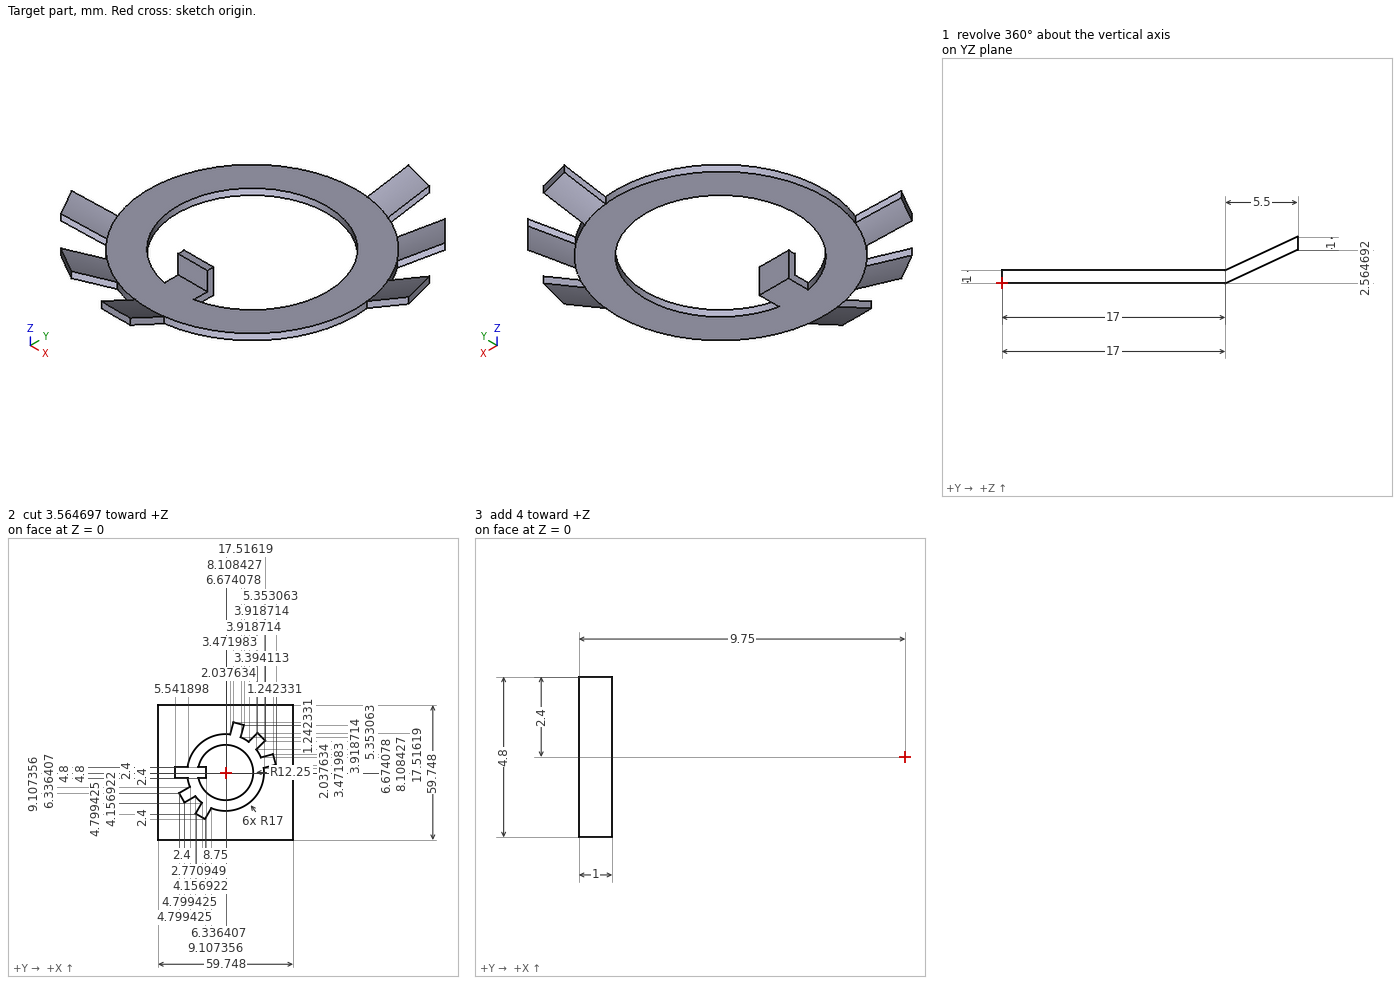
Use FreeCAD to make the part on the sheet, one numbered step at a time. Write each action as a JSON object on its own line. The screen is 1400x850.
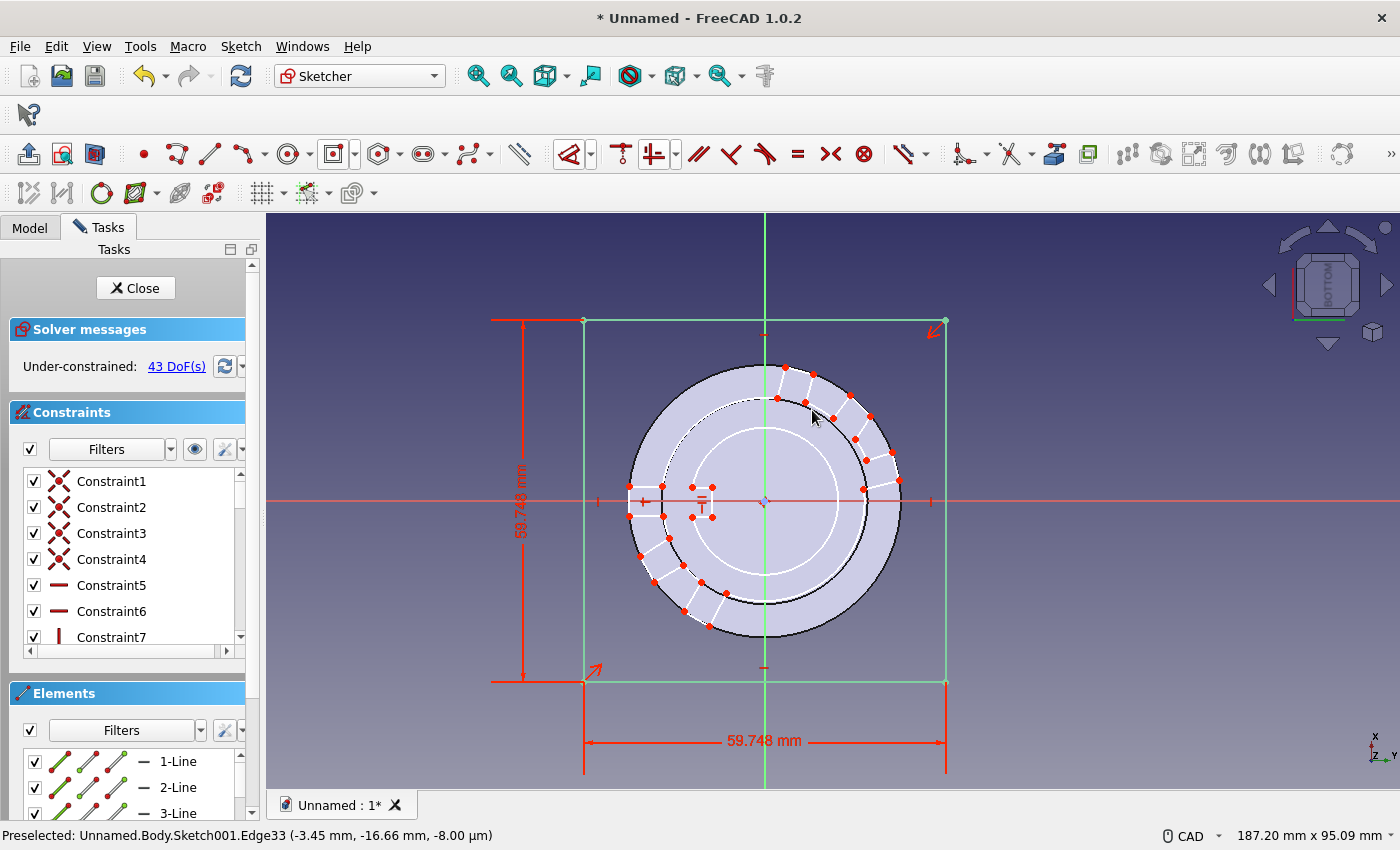
{"action": "scroll", "coordinate": [689, 571], "scroll_direction": "up", "scroll_amount": 4}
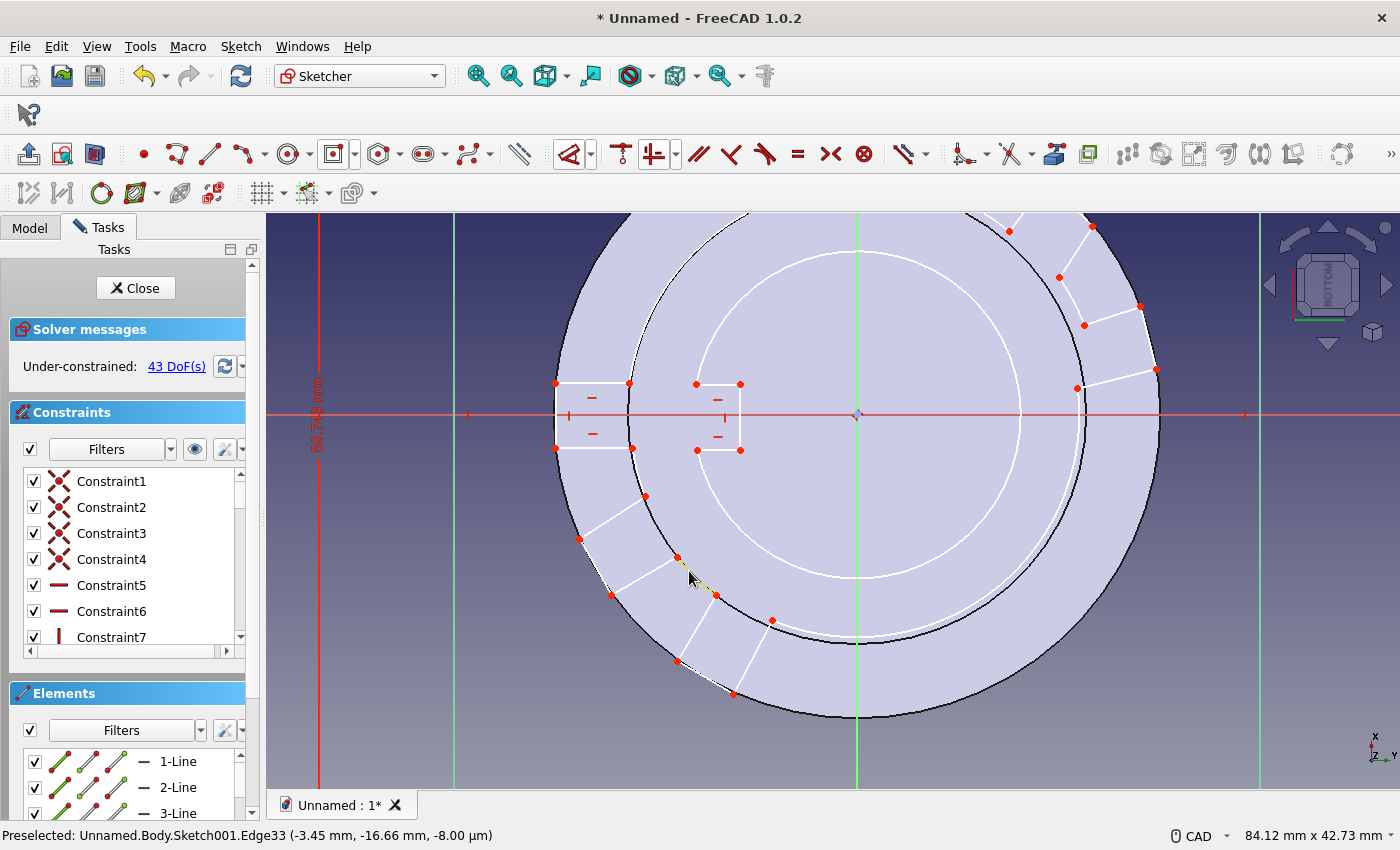
{"action": "left_click", "coordinate": [688, 570]}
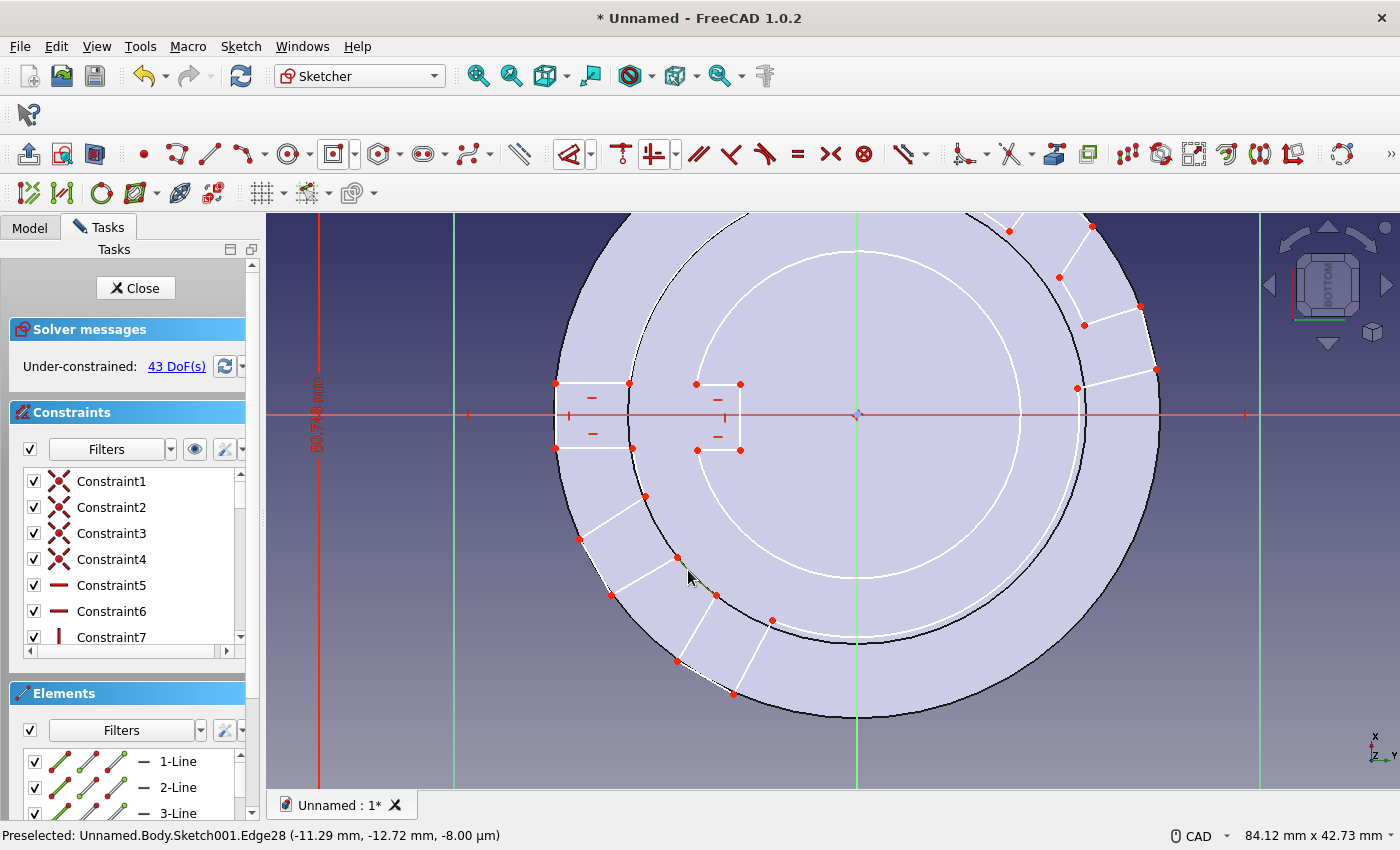
{"action": "left_click", "coordinate": [908, 631]}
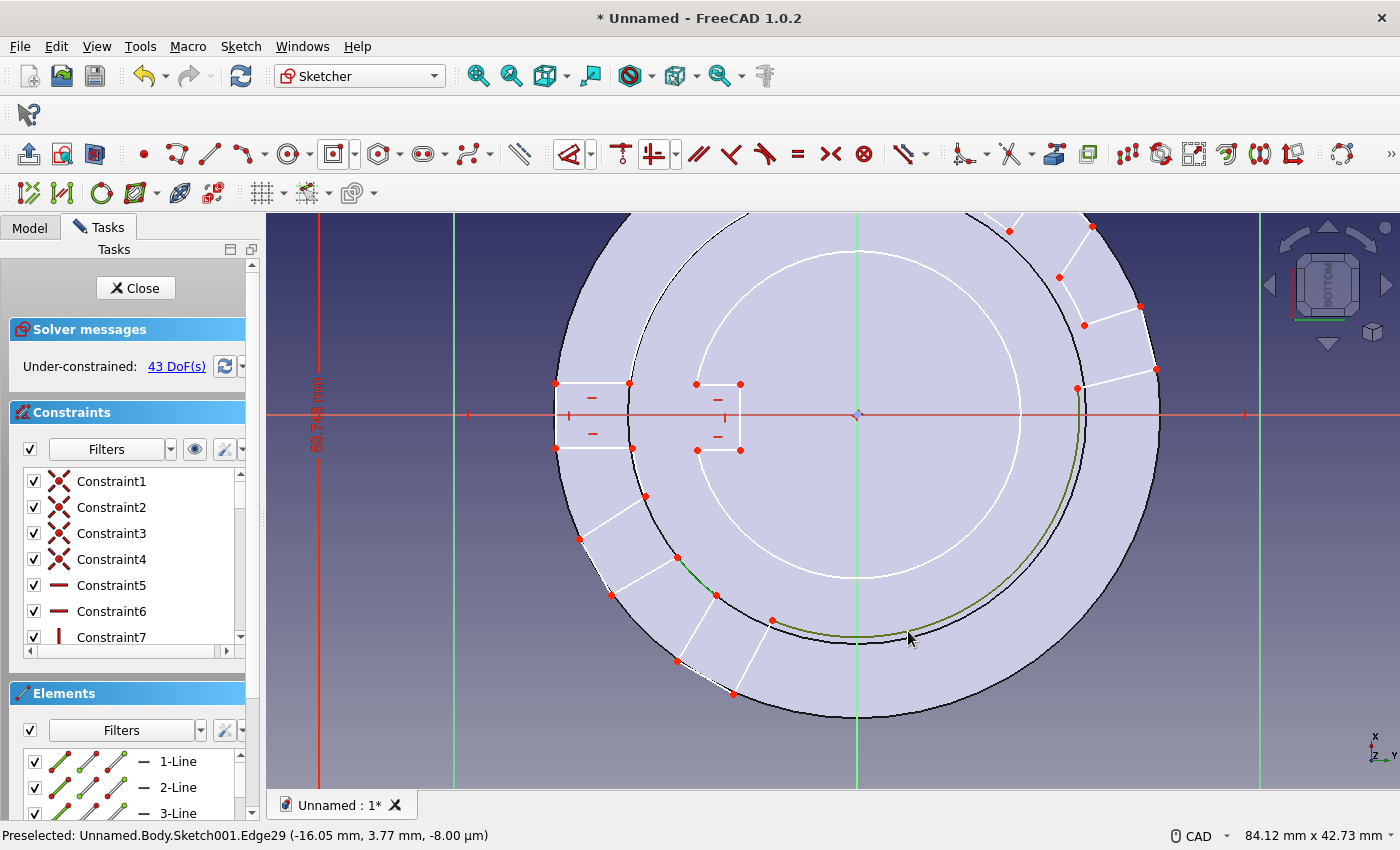
{"action": "left_click", "coordinate": [1078, 310]}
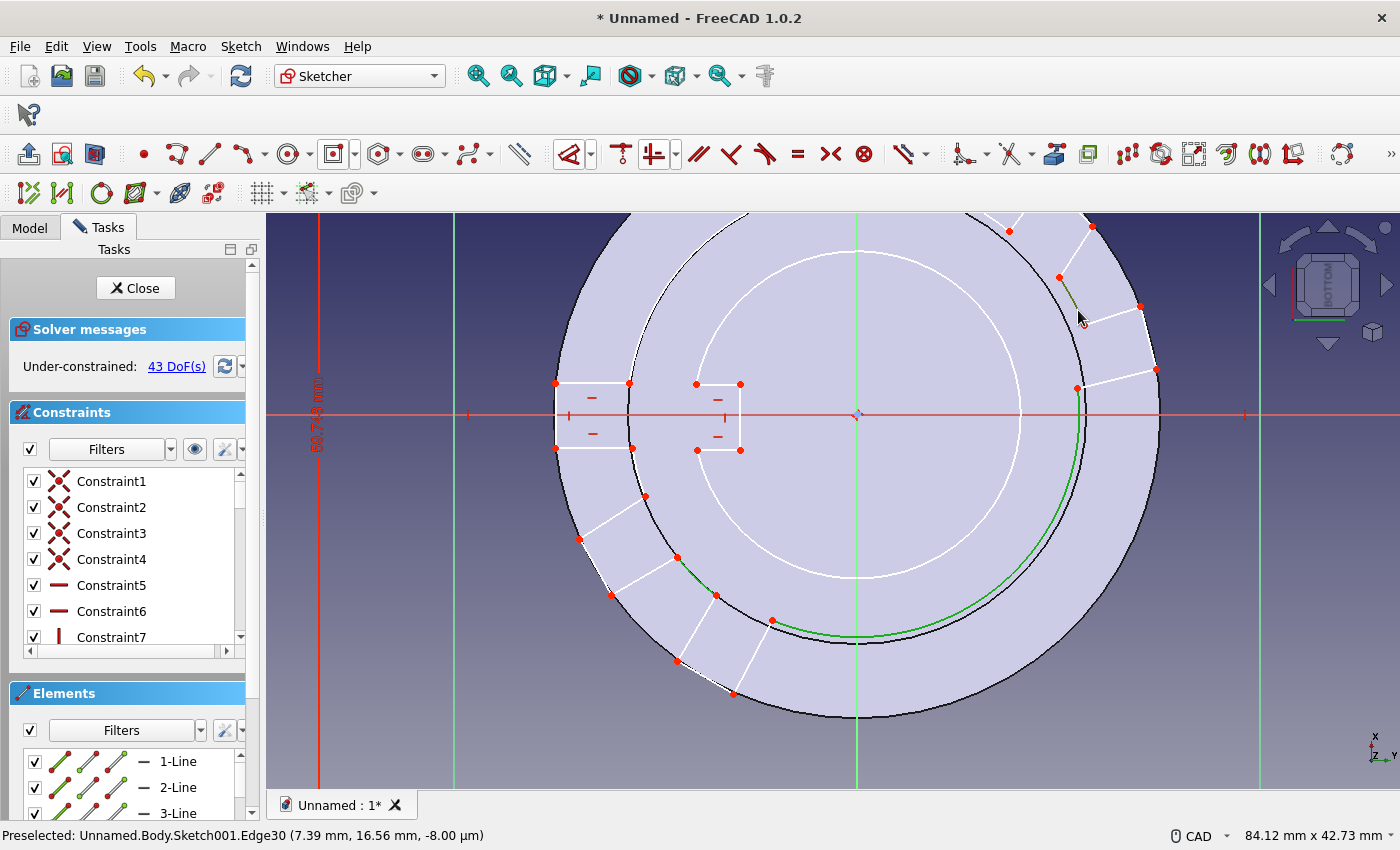
{"action": "scroll", "coordinate": [689, 571], "scroll_direction": "down", "scroll_amount": 4}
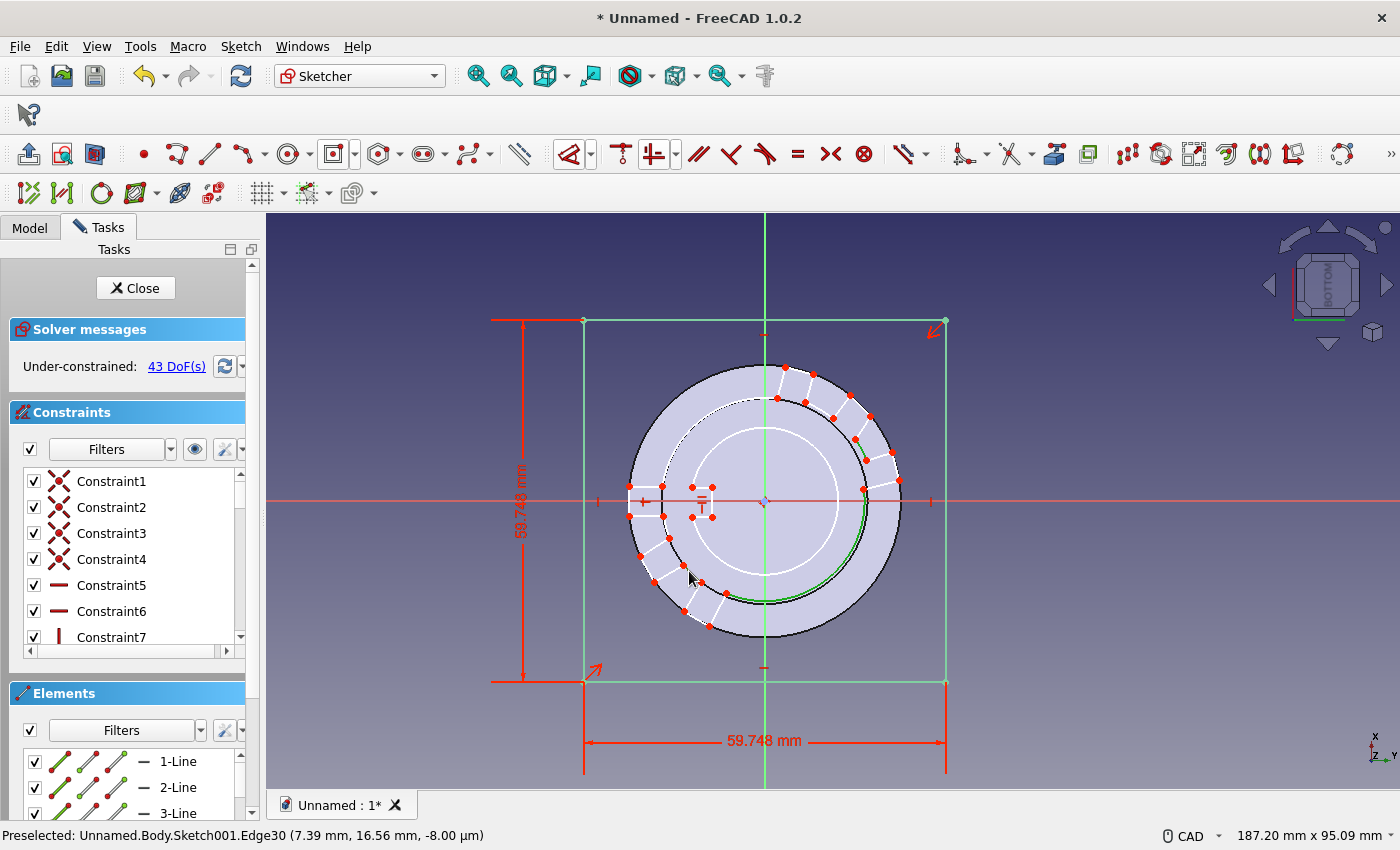
{"action": "scroll", "coordinate": [826, 413], "scroll_direction": "up", "scroll_amount": 2}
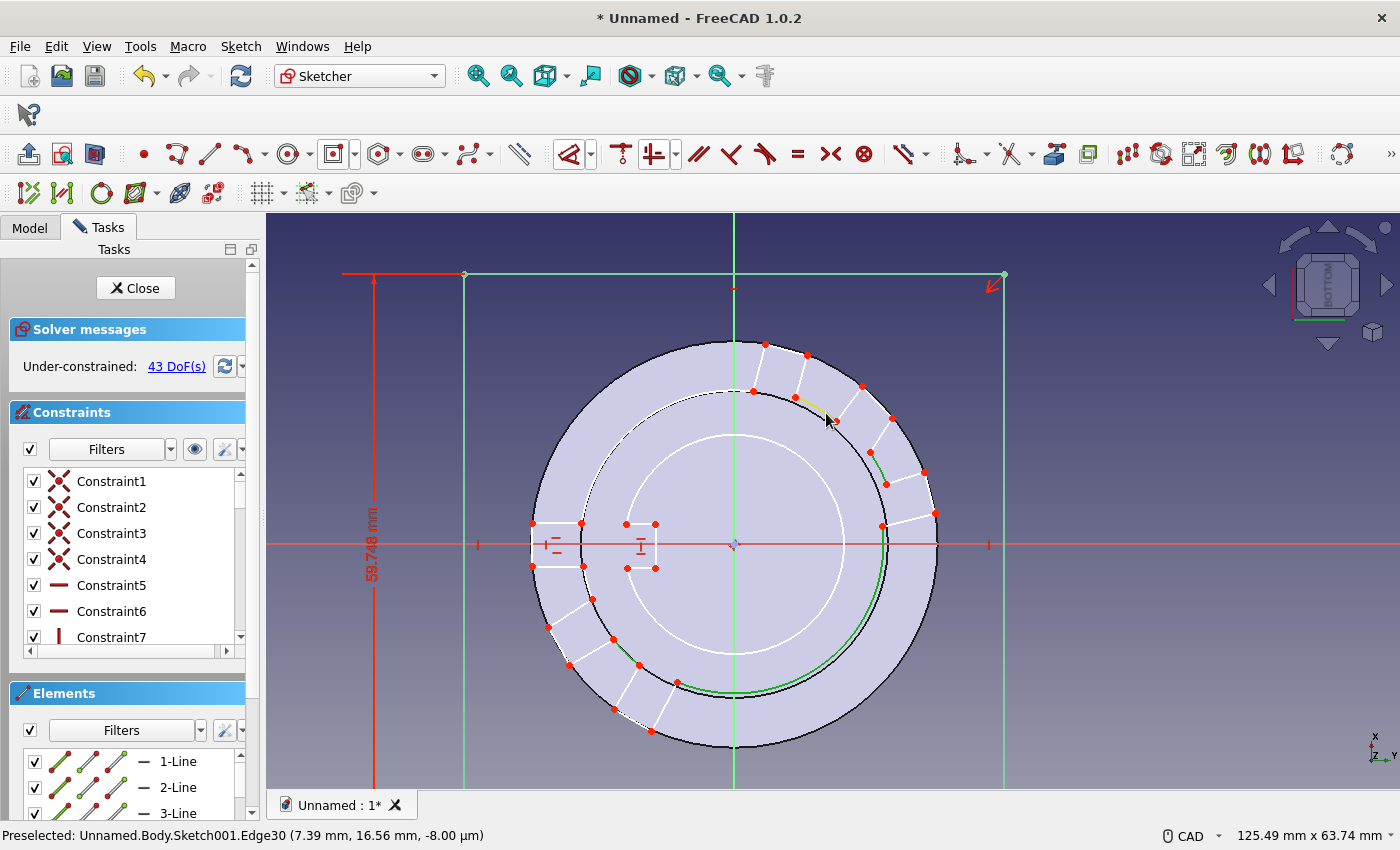
{"action": "left_click", "coordinate": [825, 413]}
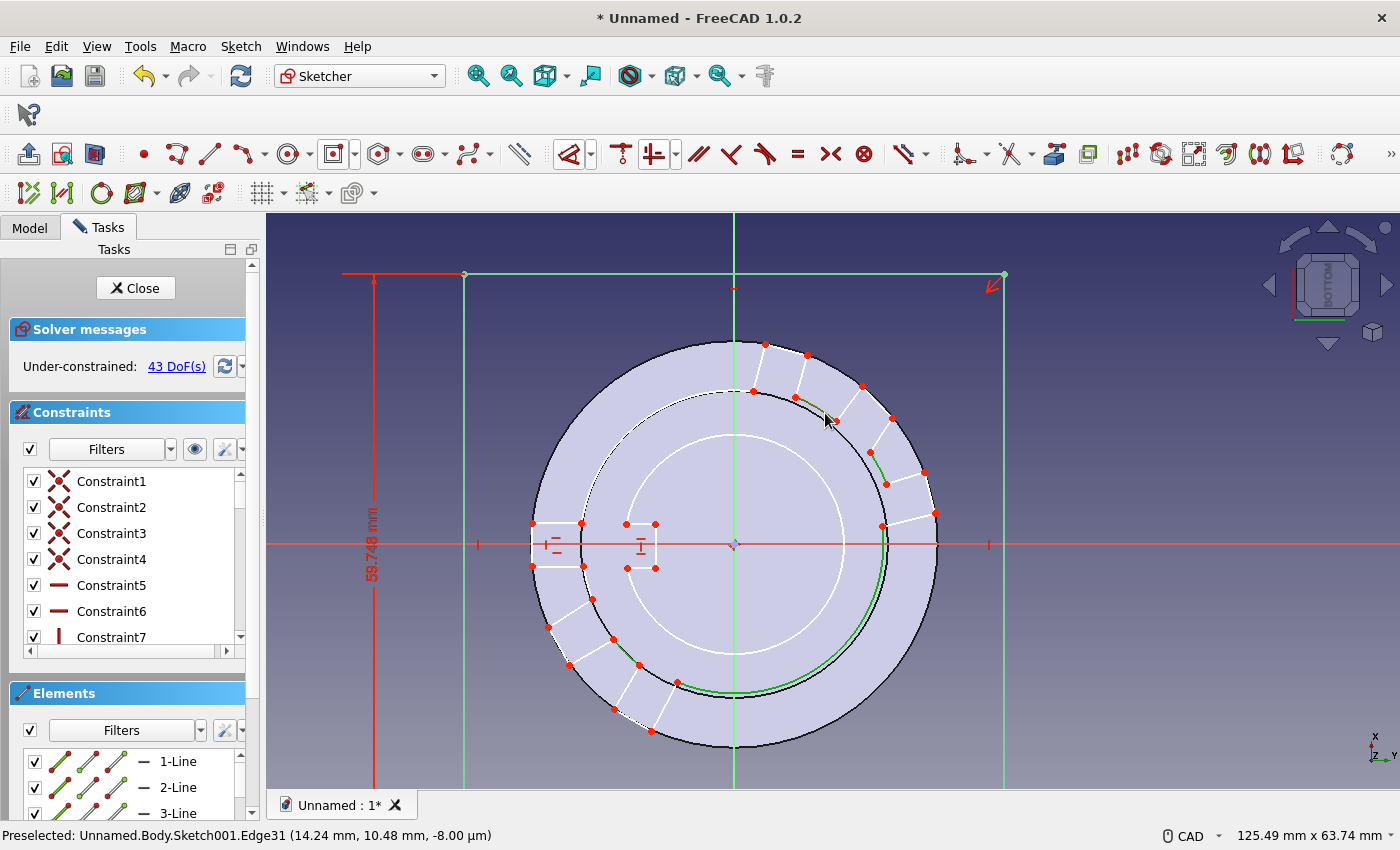
{"action": "left_click", "coordinate": [682, 399]}